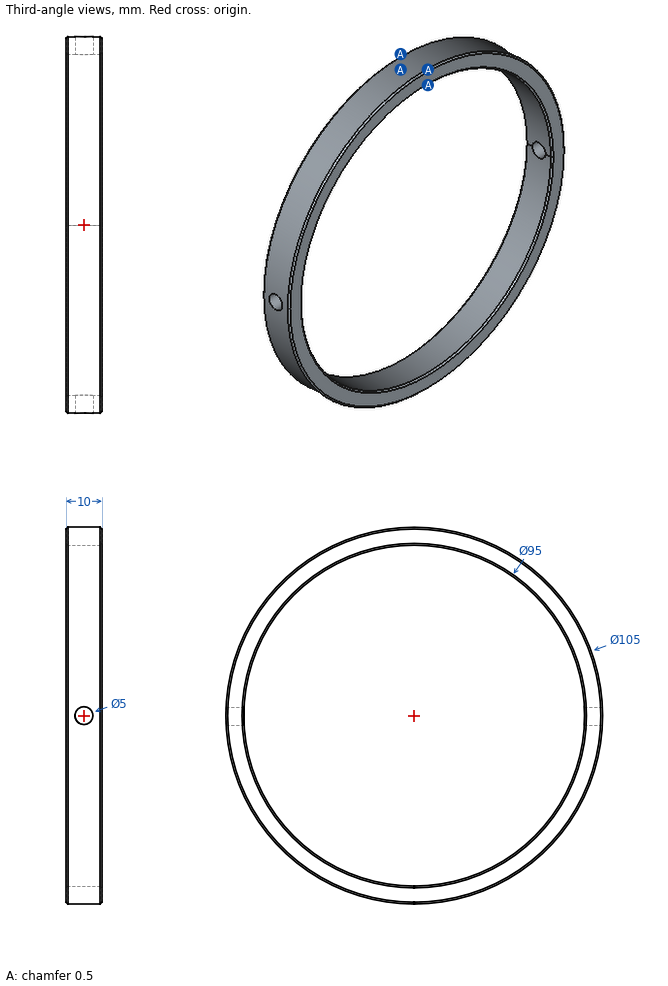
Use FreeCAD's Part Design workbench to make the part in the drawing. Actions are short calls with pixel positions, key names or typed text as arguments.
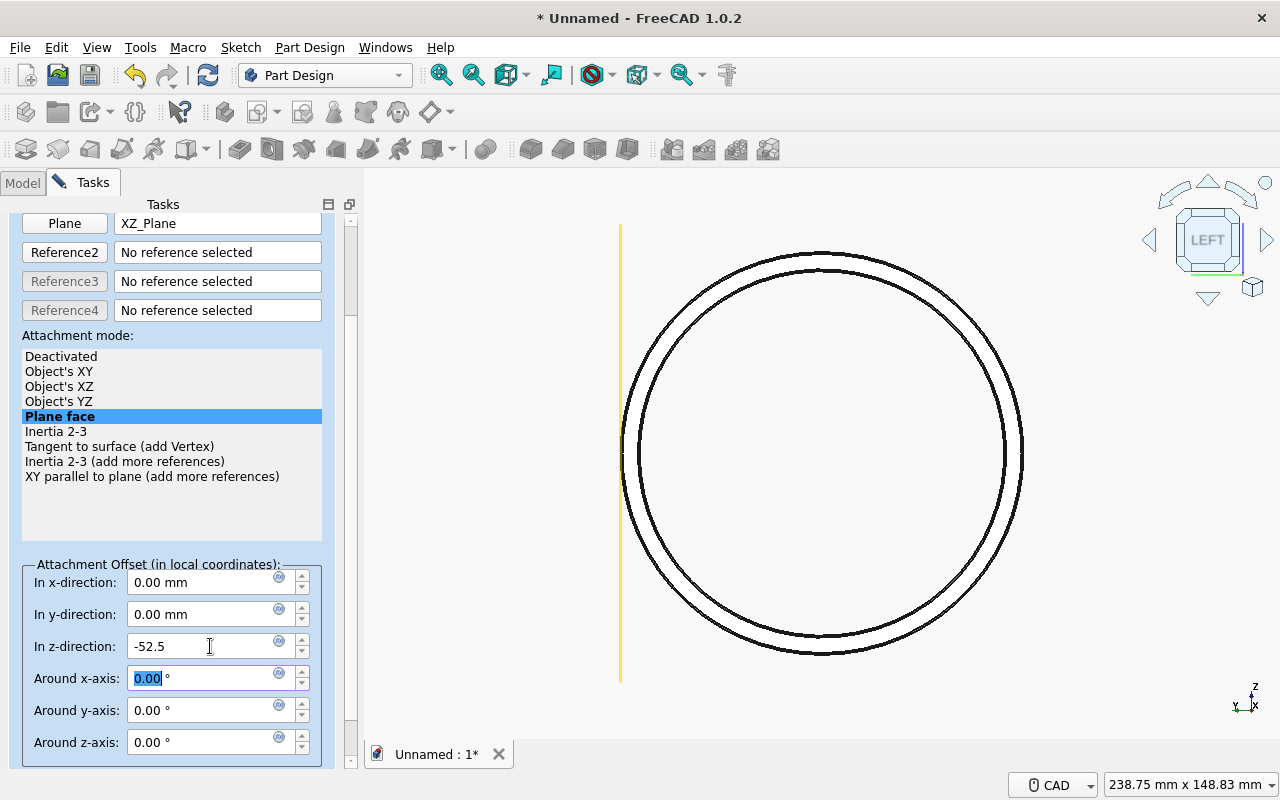
scroll(351, 491, up, 3)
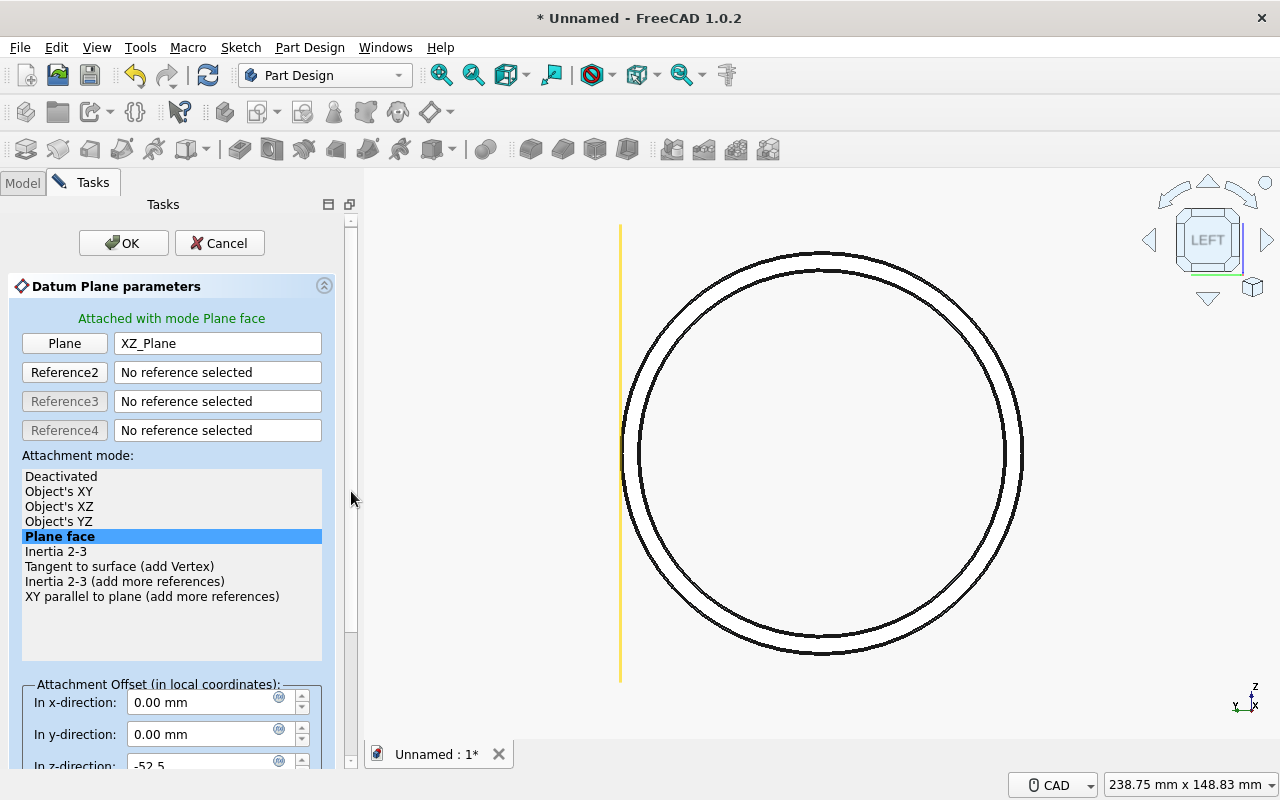
click(124, 243)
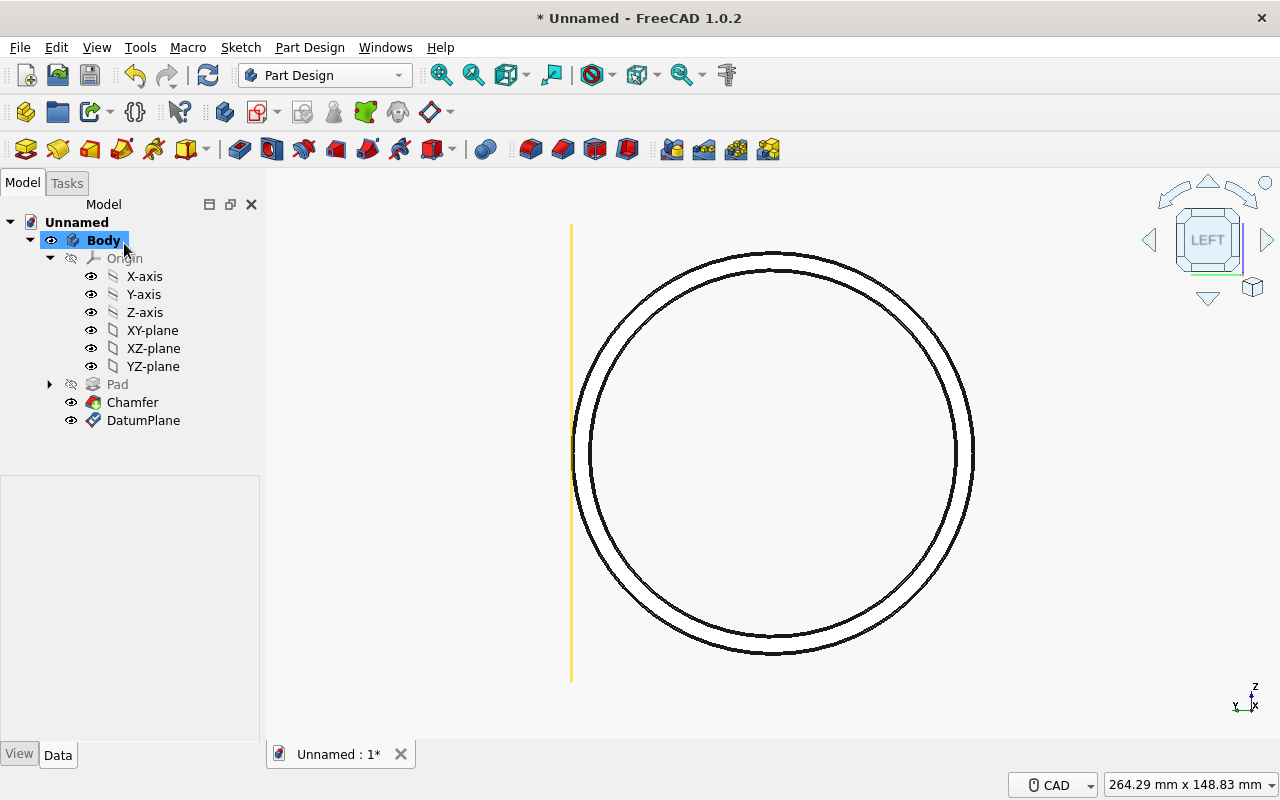
click(116, 420)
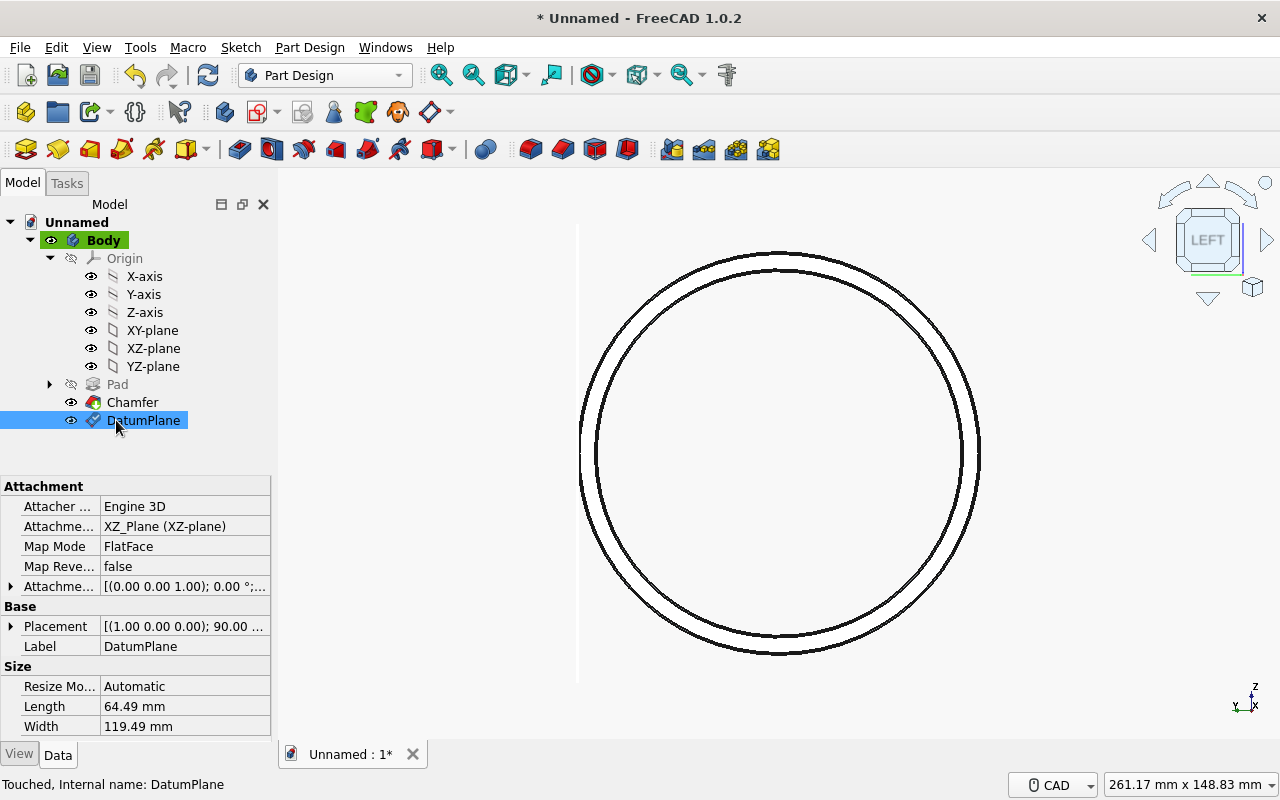
click(258, 112)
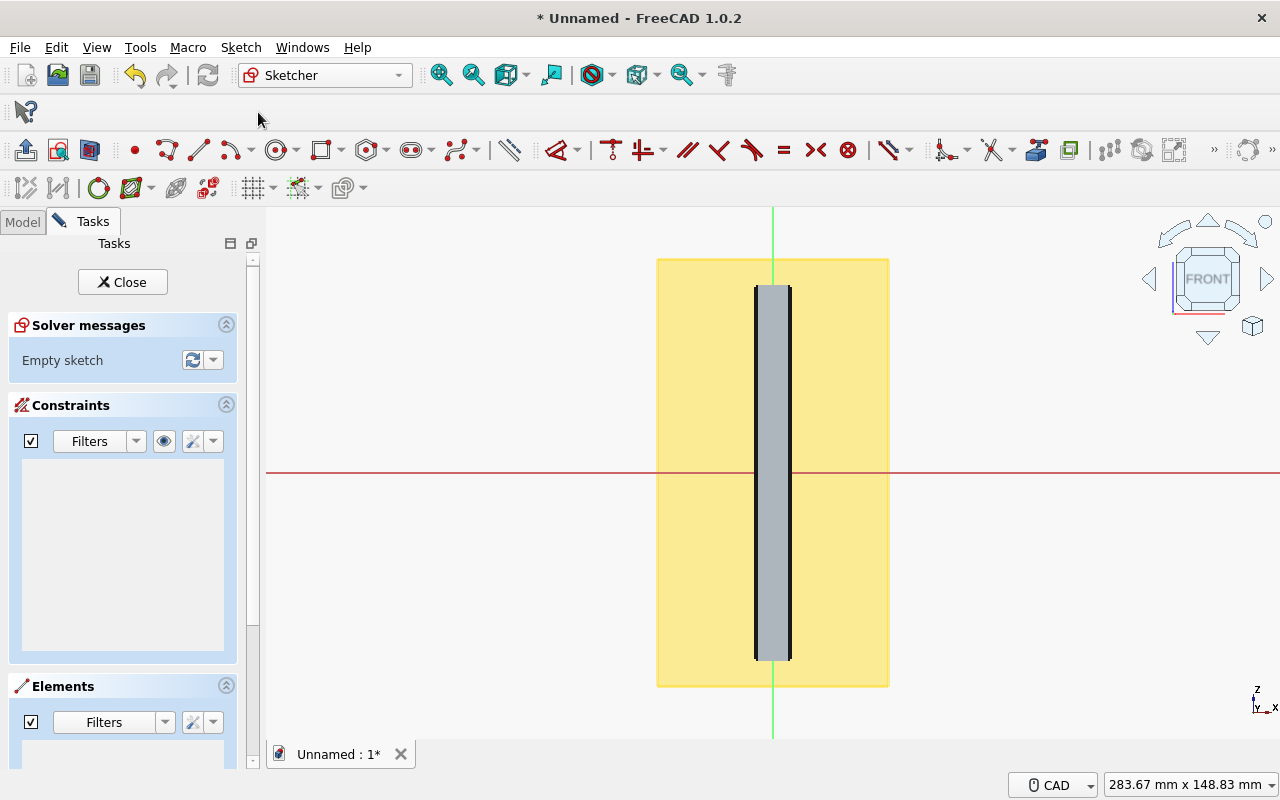
click(90, 150)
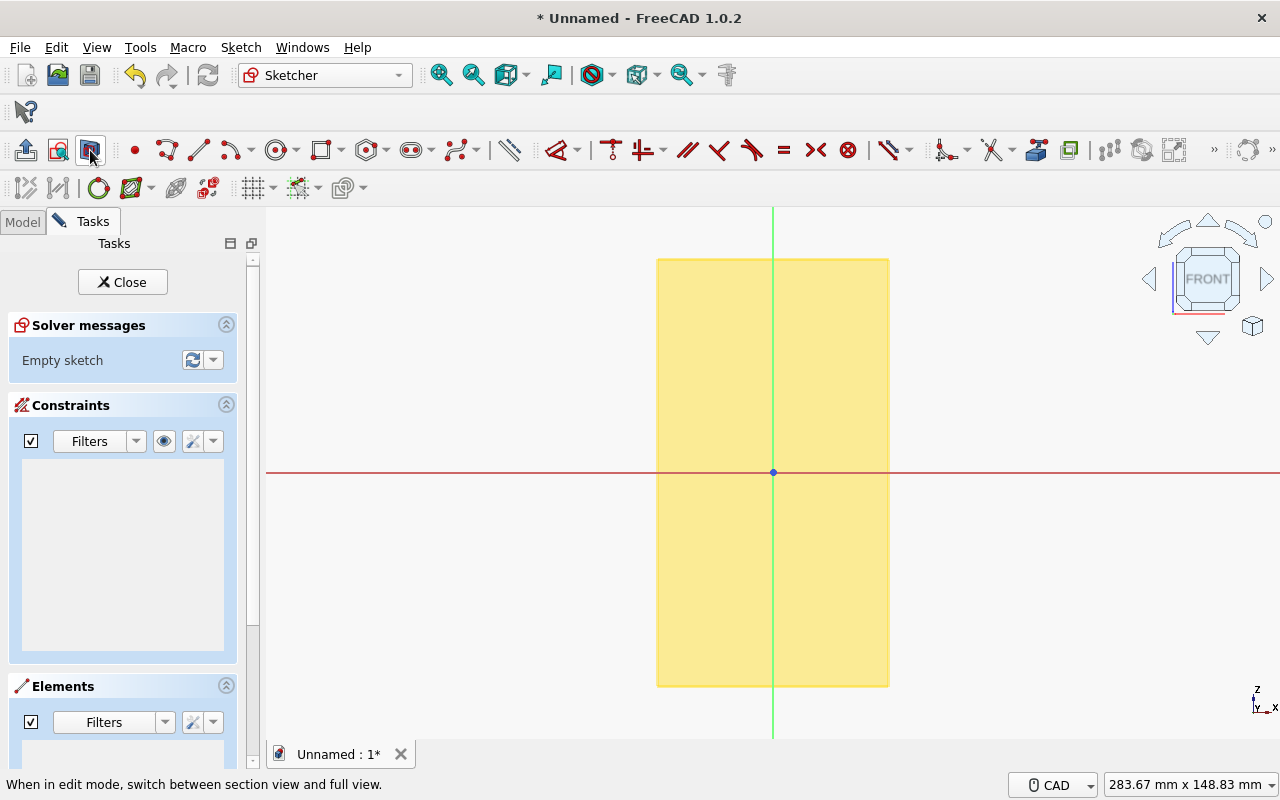
scroll(777, 473, up, 15)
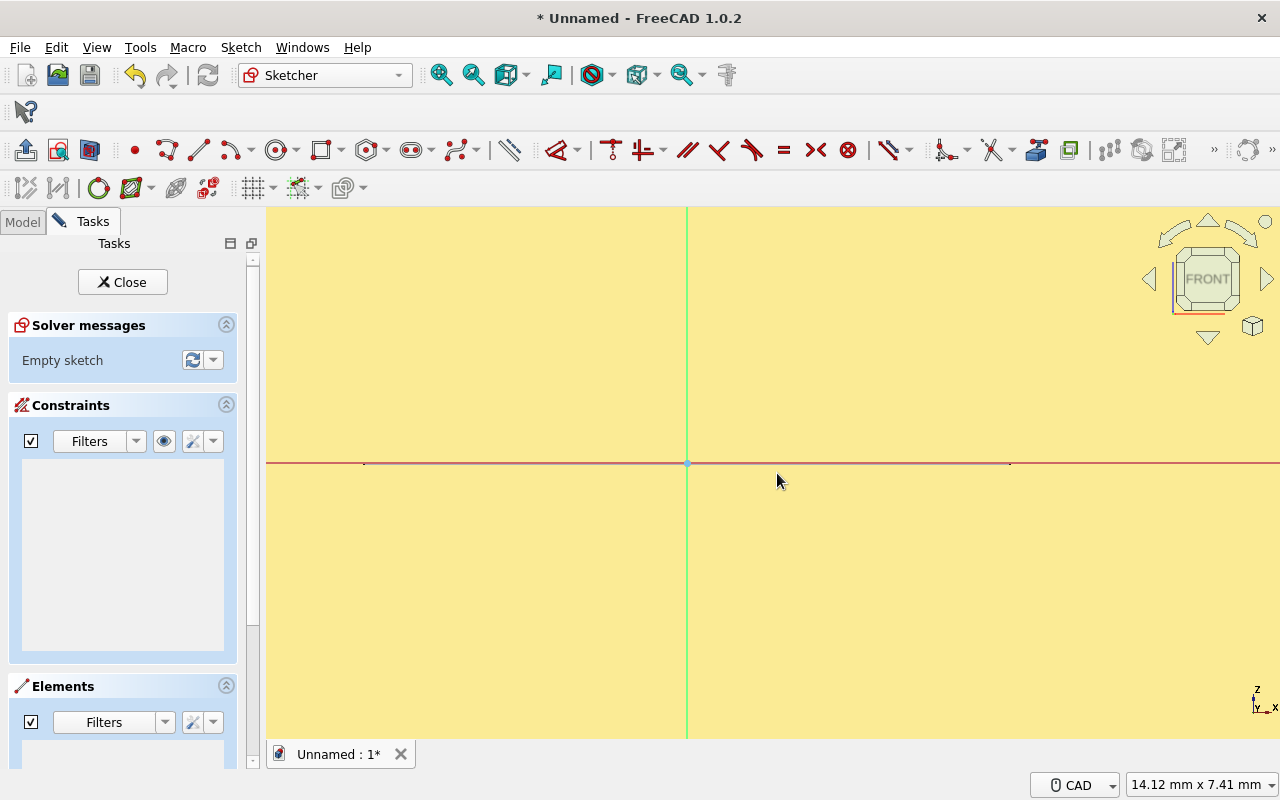
click(276, 150)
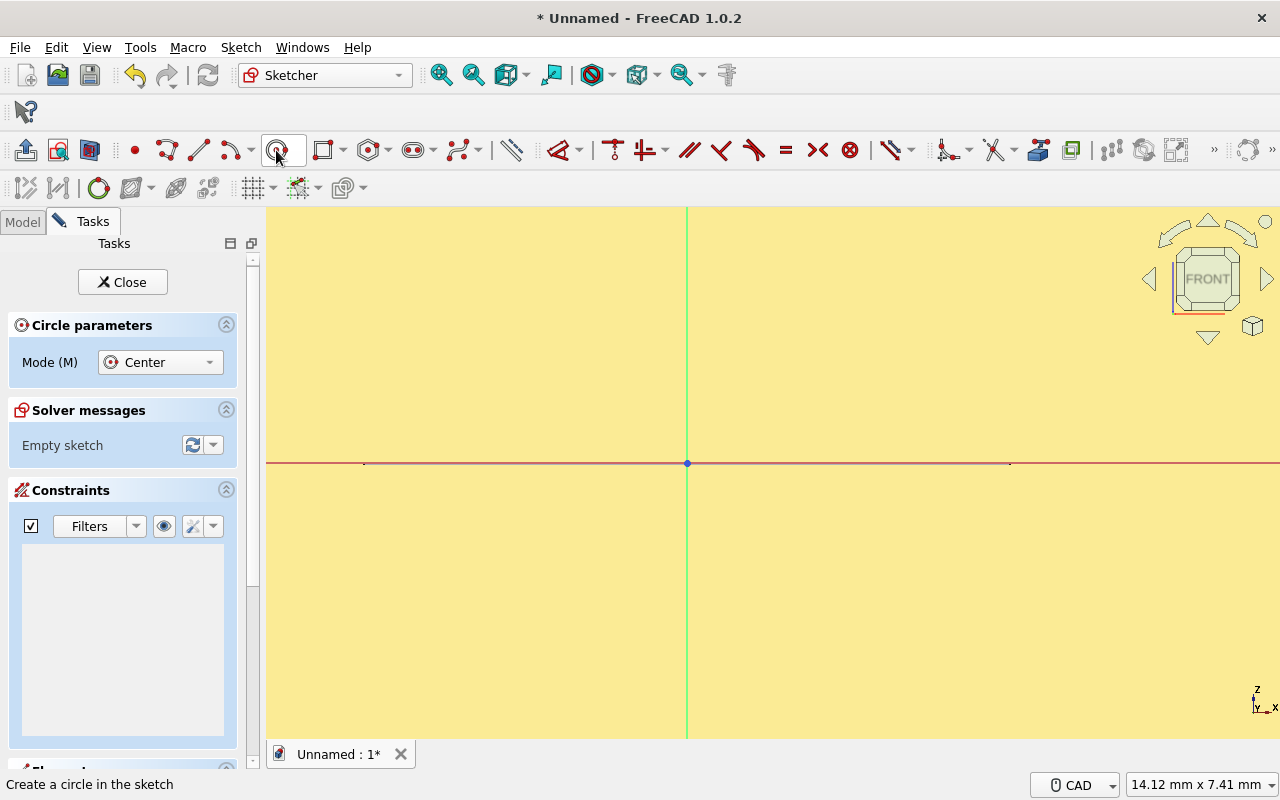
click(687, 463)
click(814, 337)
key(Escape)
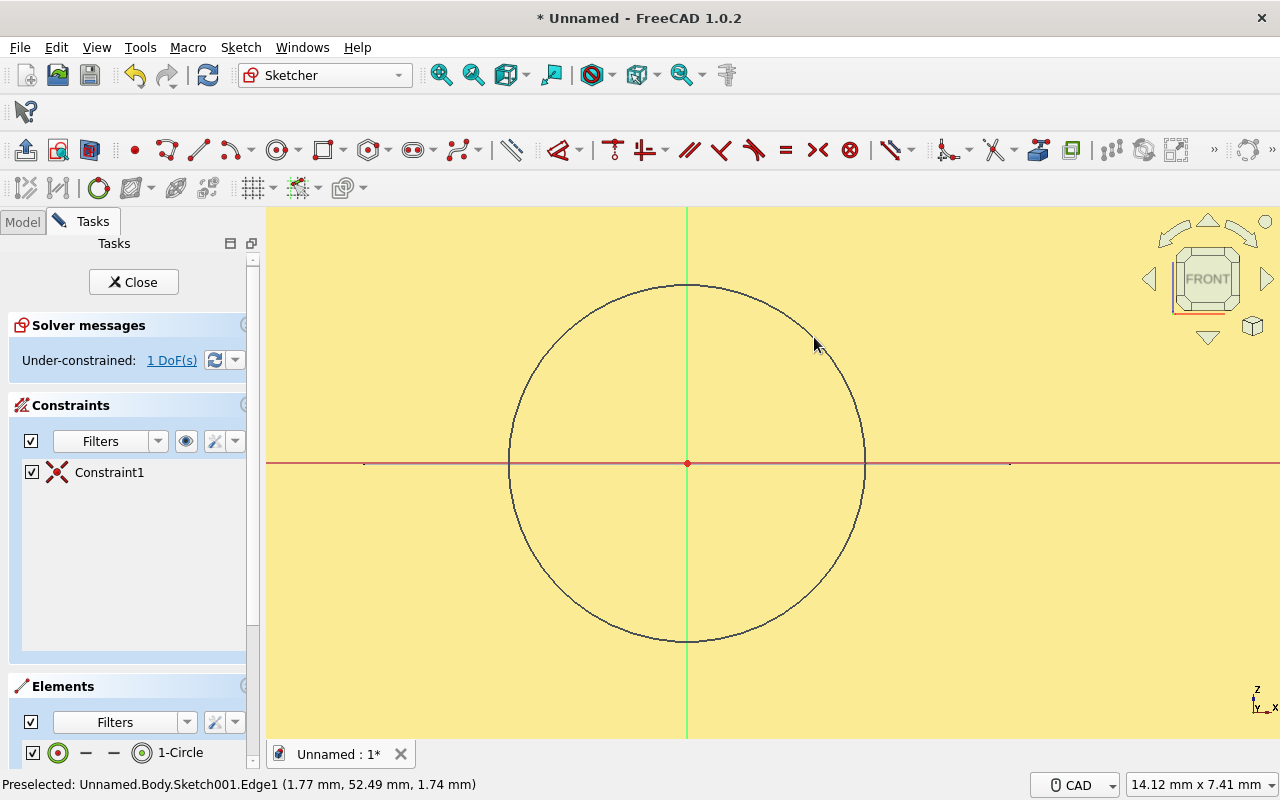
click(558, 150)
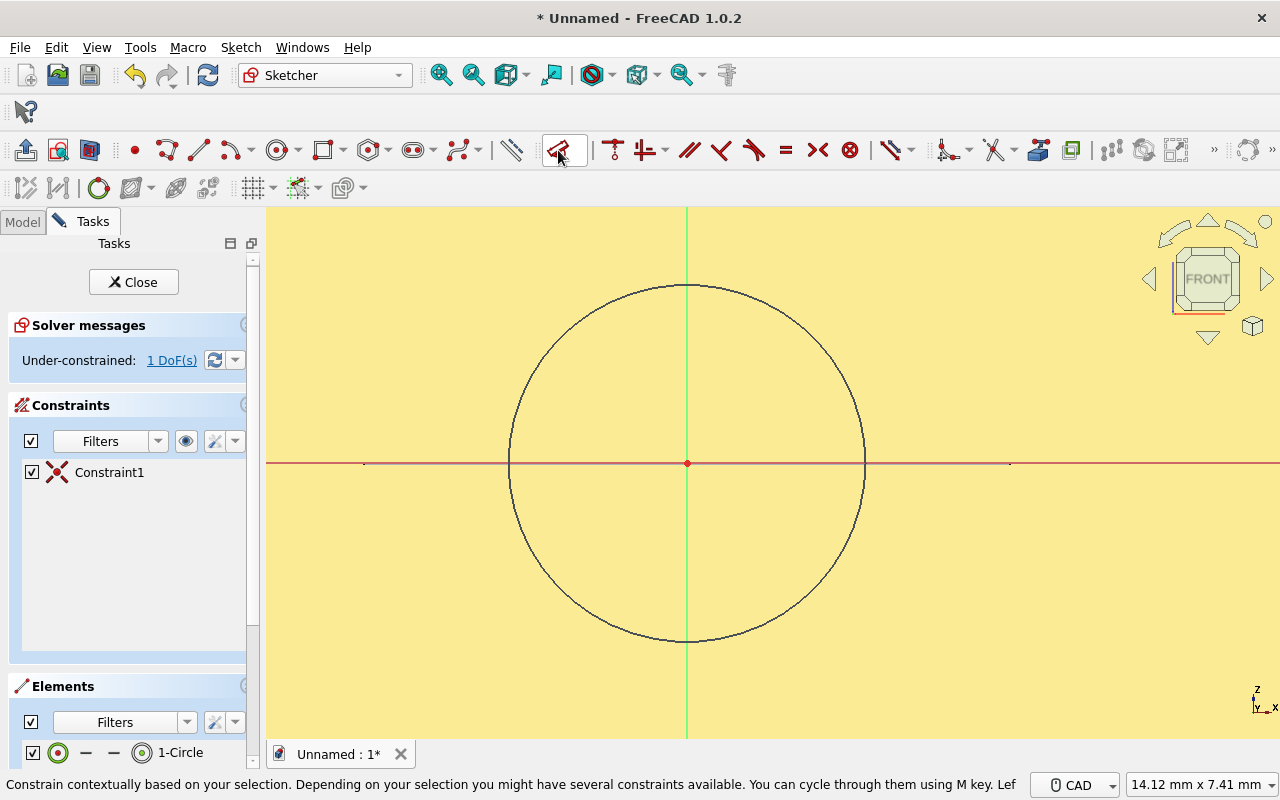
click(813, 337)
click(836, 314)